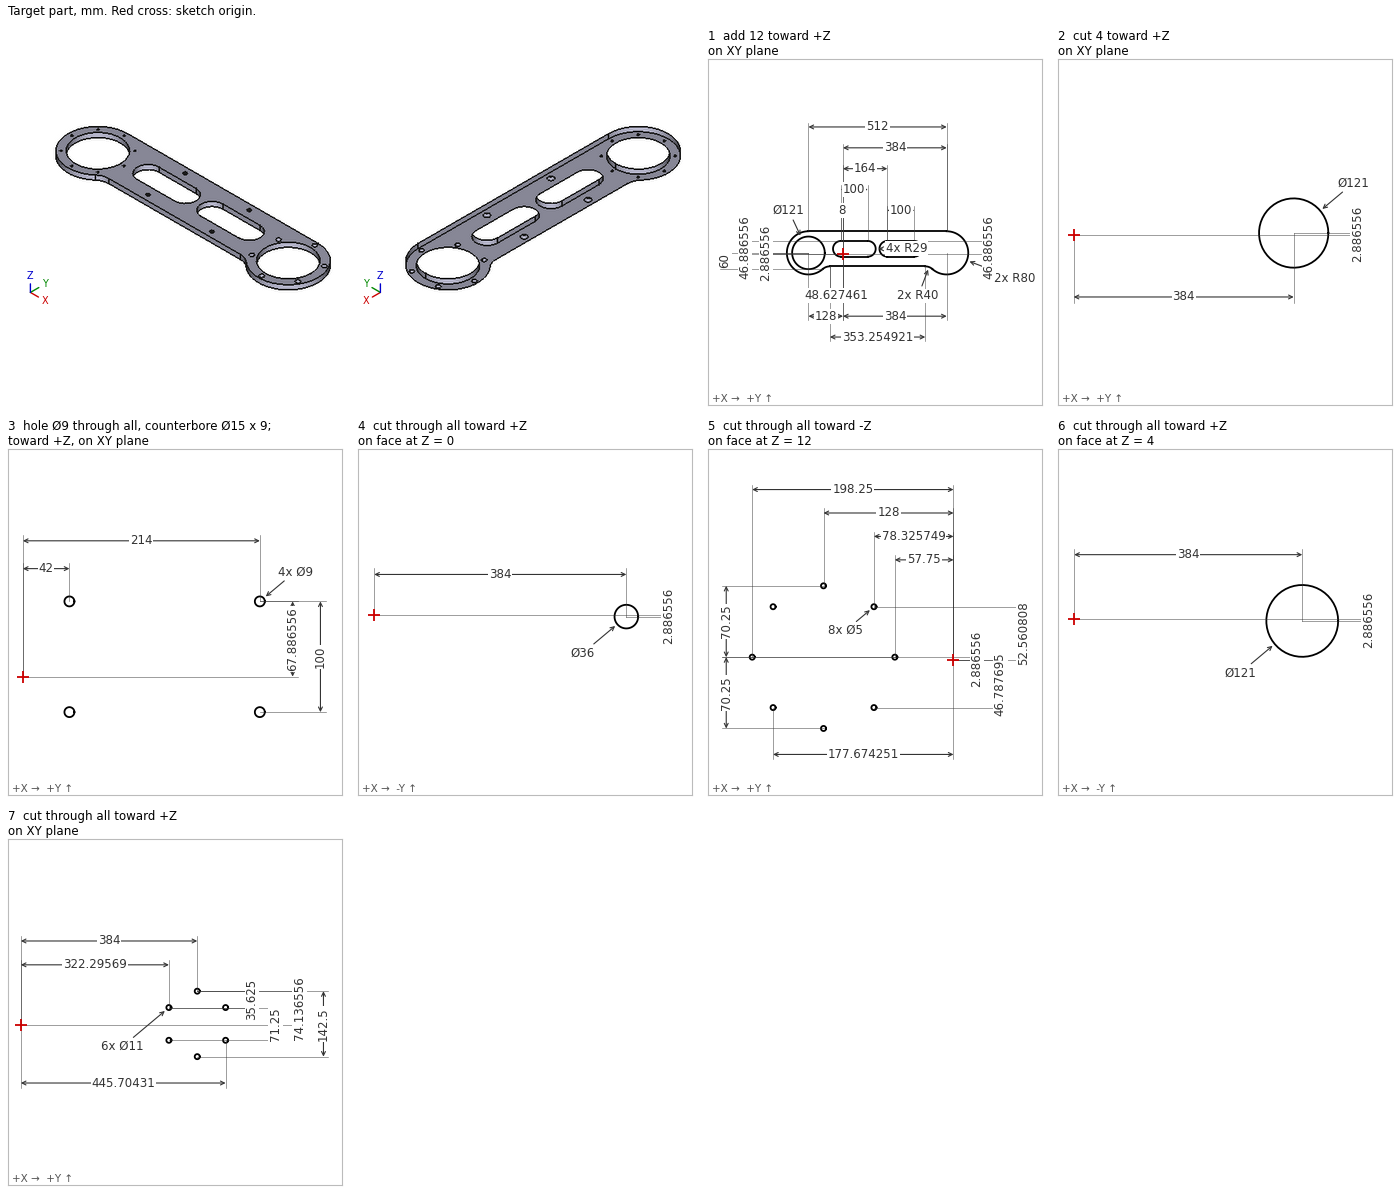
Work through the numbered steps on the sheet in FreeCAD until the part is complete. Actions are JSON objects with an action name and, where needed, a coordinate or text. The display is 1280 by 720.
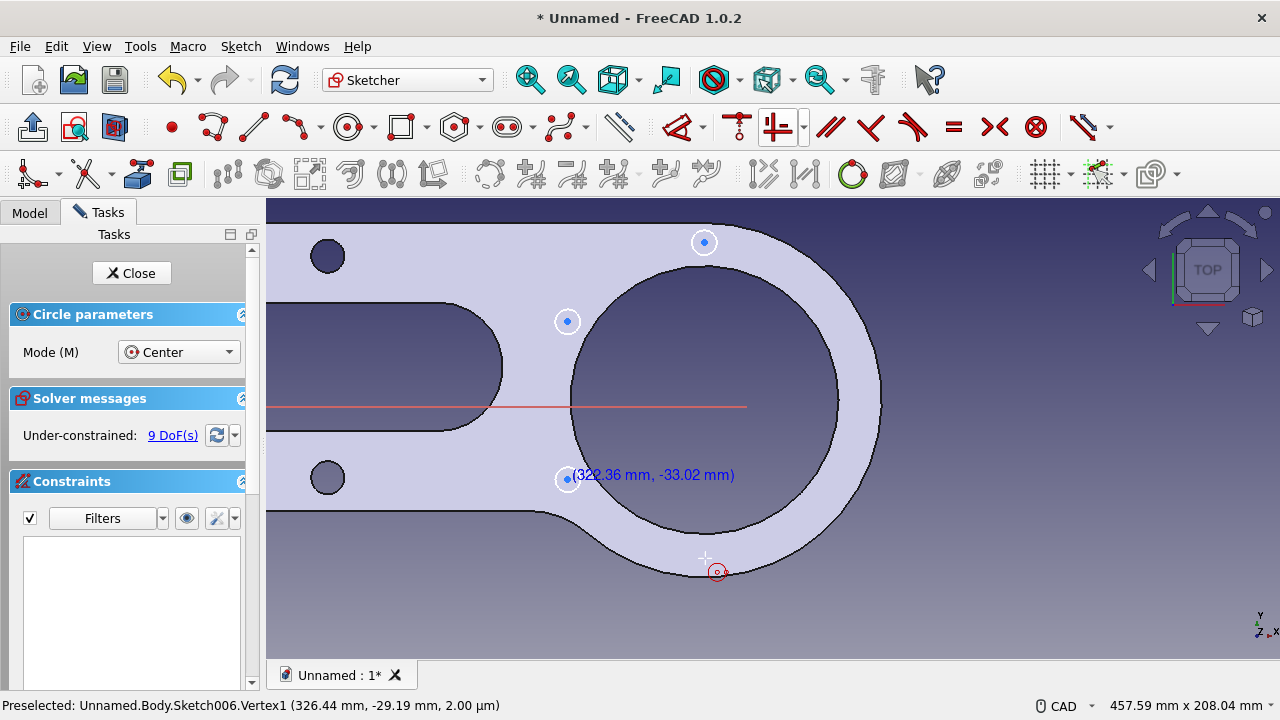
{"action": "left_click", "coordinate": [703, 557]}
{"action": "left_click", "coordinate": [723, 538]}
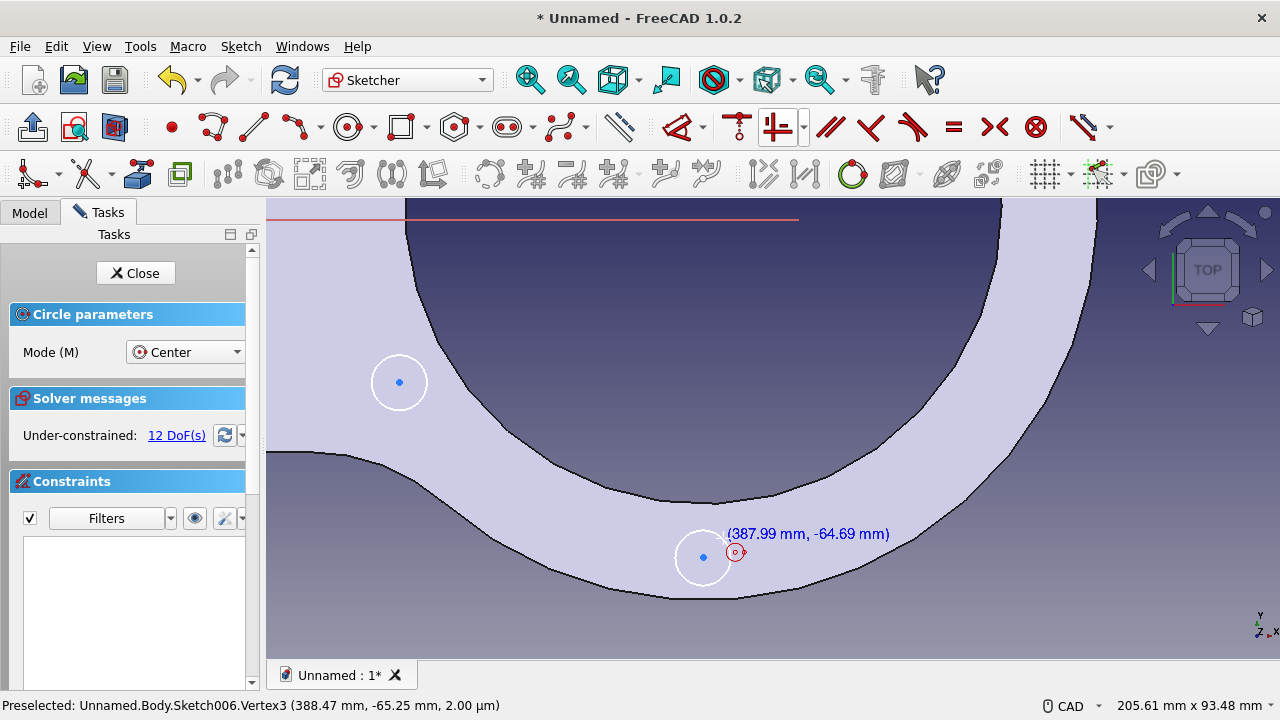
{"action": "left_click", "coordinate": [1008, 381]}
{"action": "left_click", "coordinate": [1027, 362]}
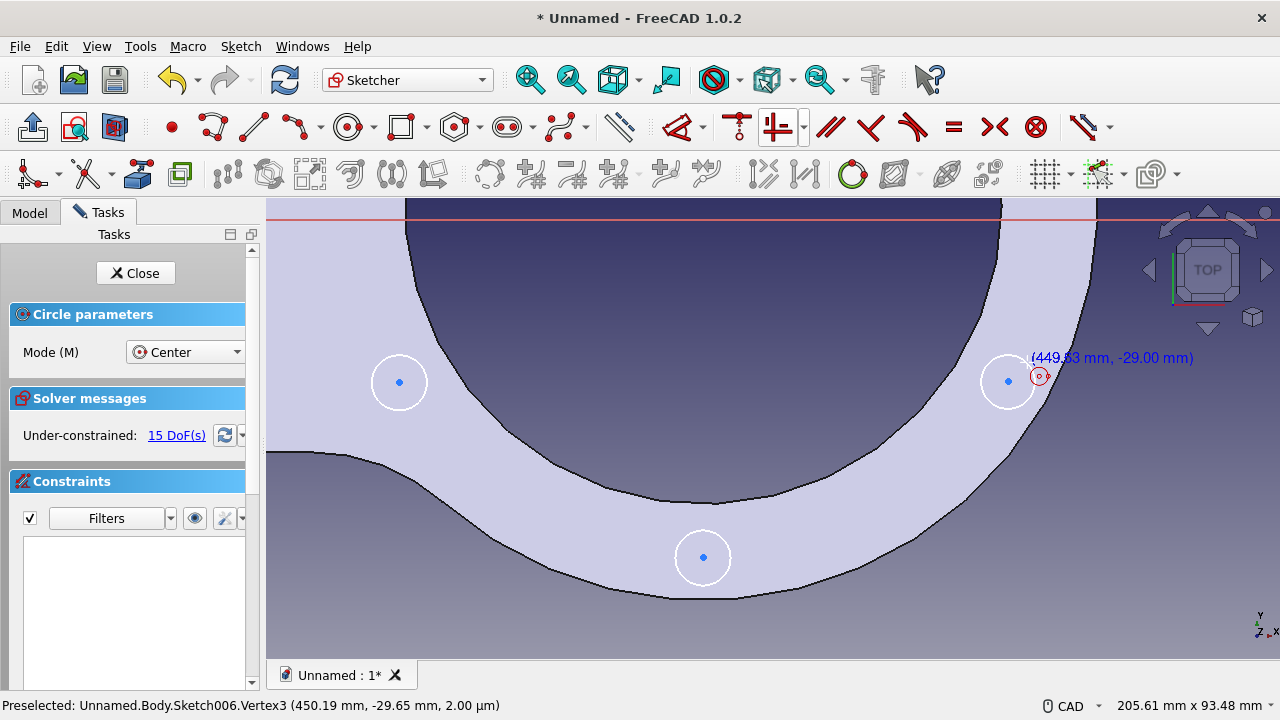
{"action": "scroll", "coordinate": [705, 558], "scroll_direction": "down", "scroll_amount": 5}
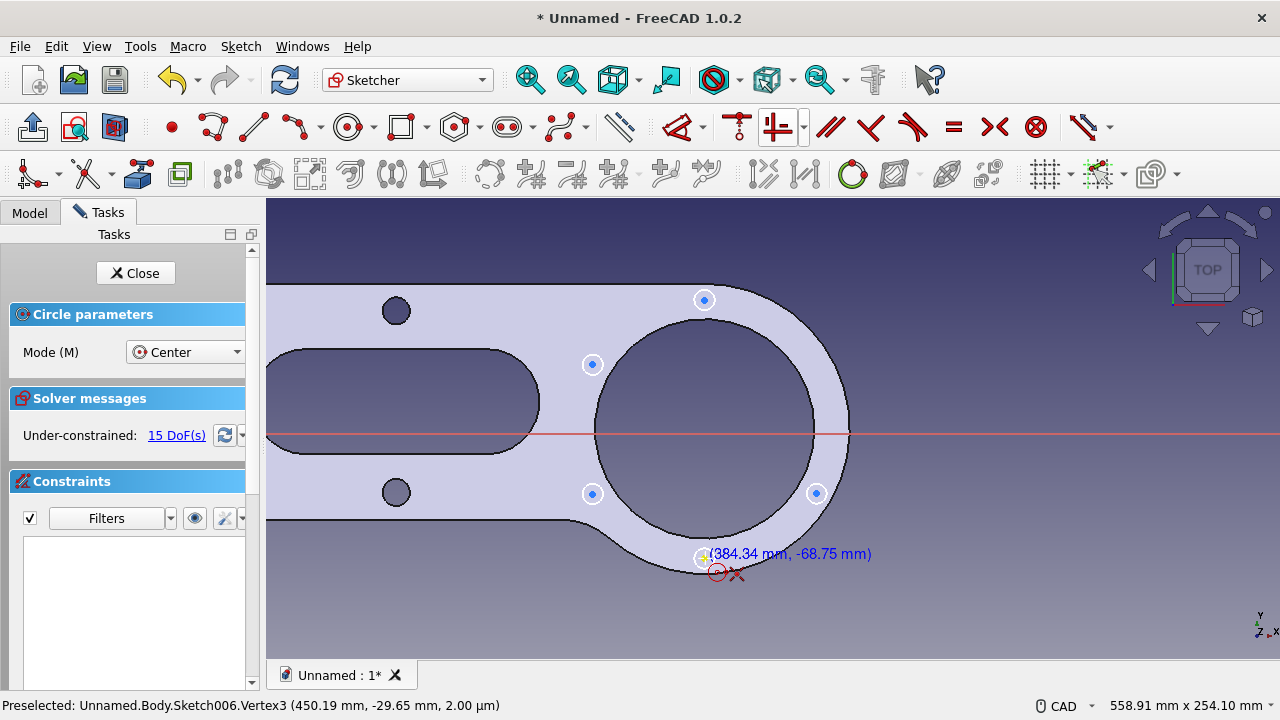
{"action": "scroll", "coordinate": [817, 364], "scroll_direction": "up", "scroll_amount": 5}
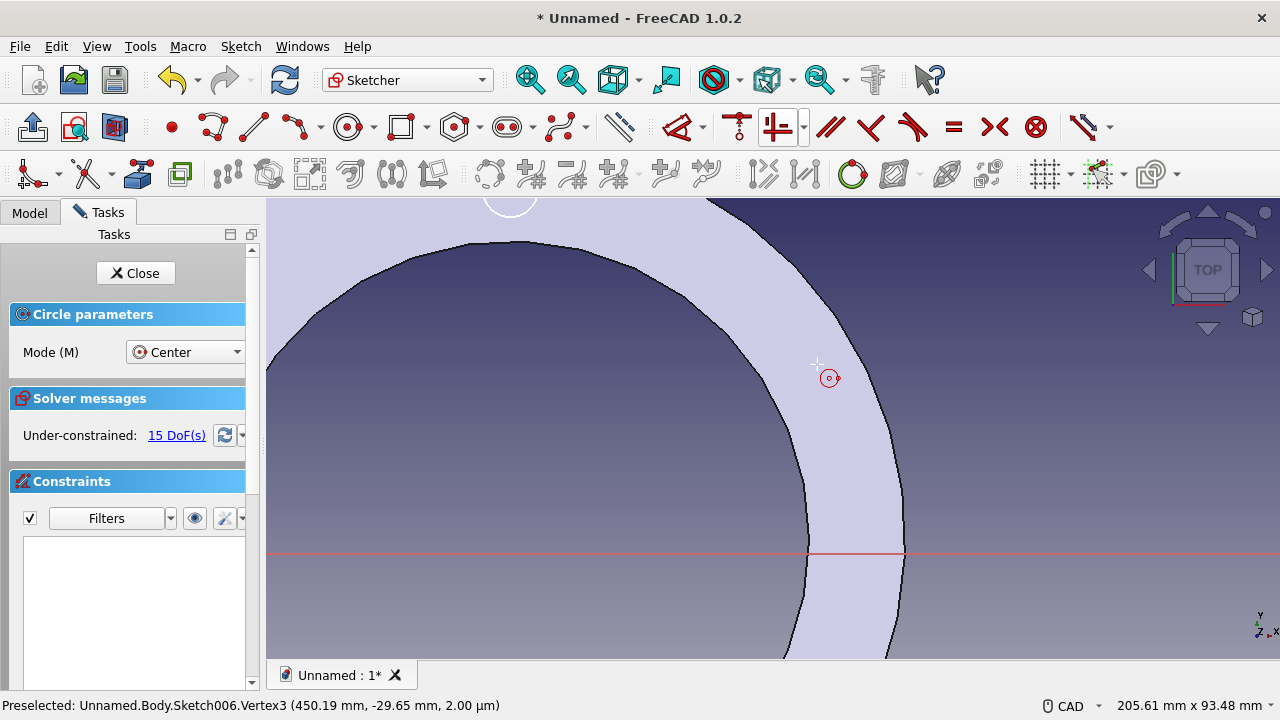
{"action": "left_click", "coordinate": [815, 364]}
{"action": "left_click", "coordinate": [834, 345]}
{"action": "key", "text": "Escape"}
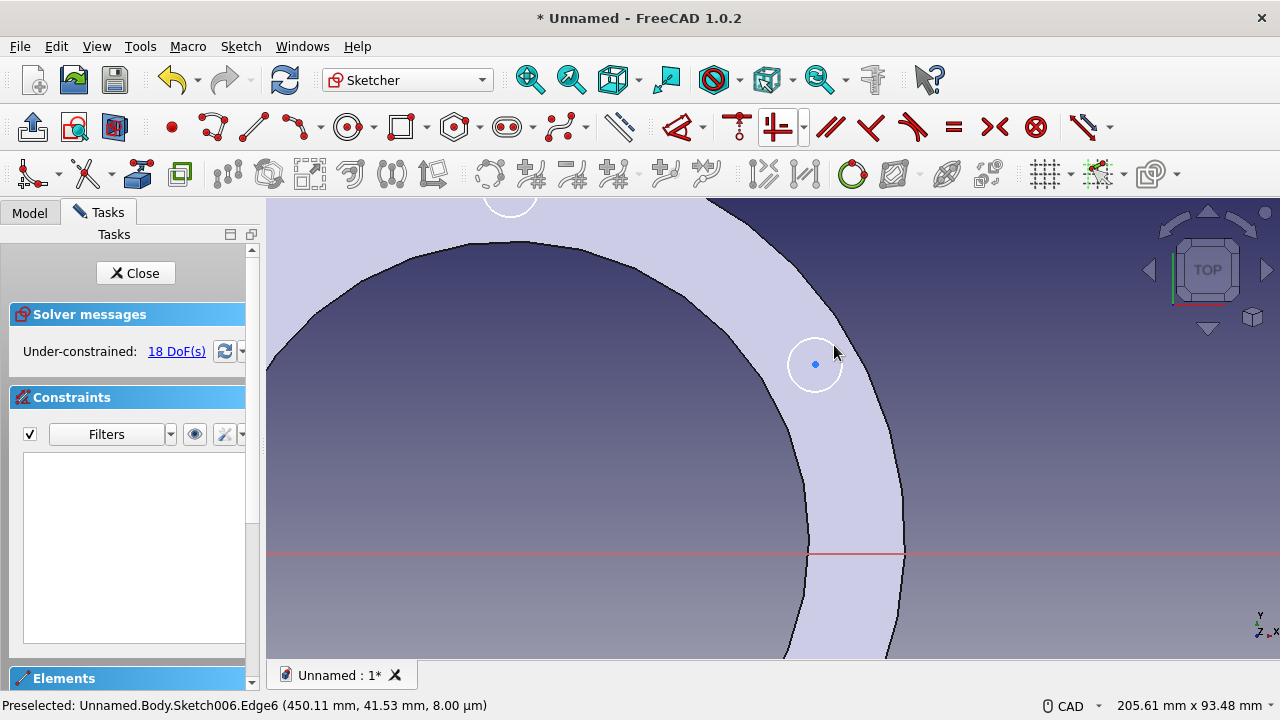
{"action": "scroll", "coordinate": [817, 364], "scroll_direction": "down", "scroll_amount": 5}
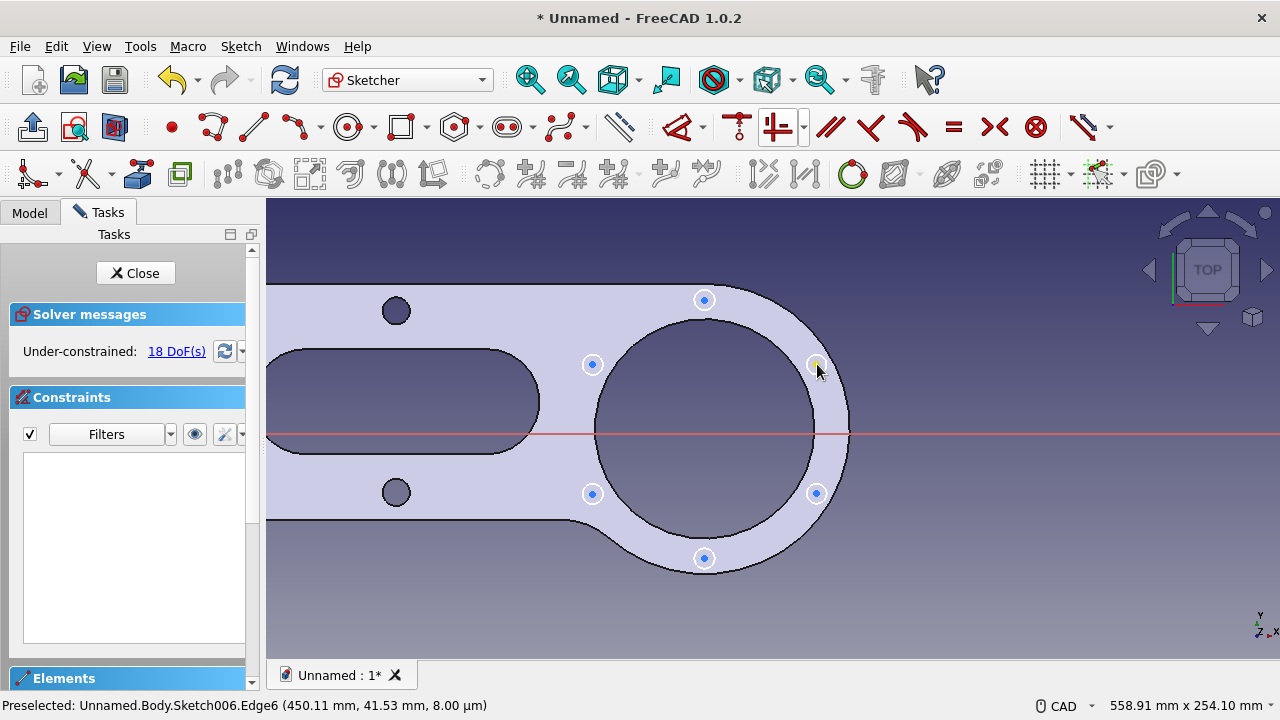
{"action": "scroll", "coordinate": [712, 293], "scroll_direction": "up", "scroll_amount": 2}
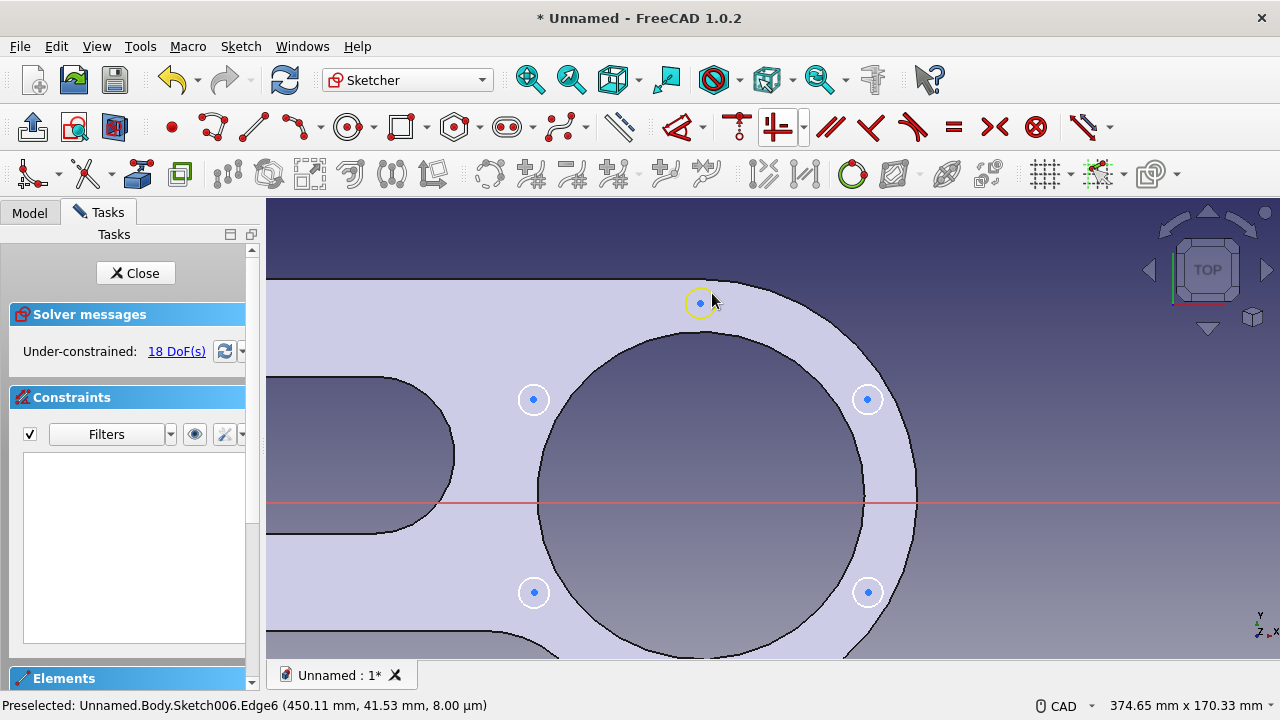
{"action": "left_click", "coordinate": [711, 293]}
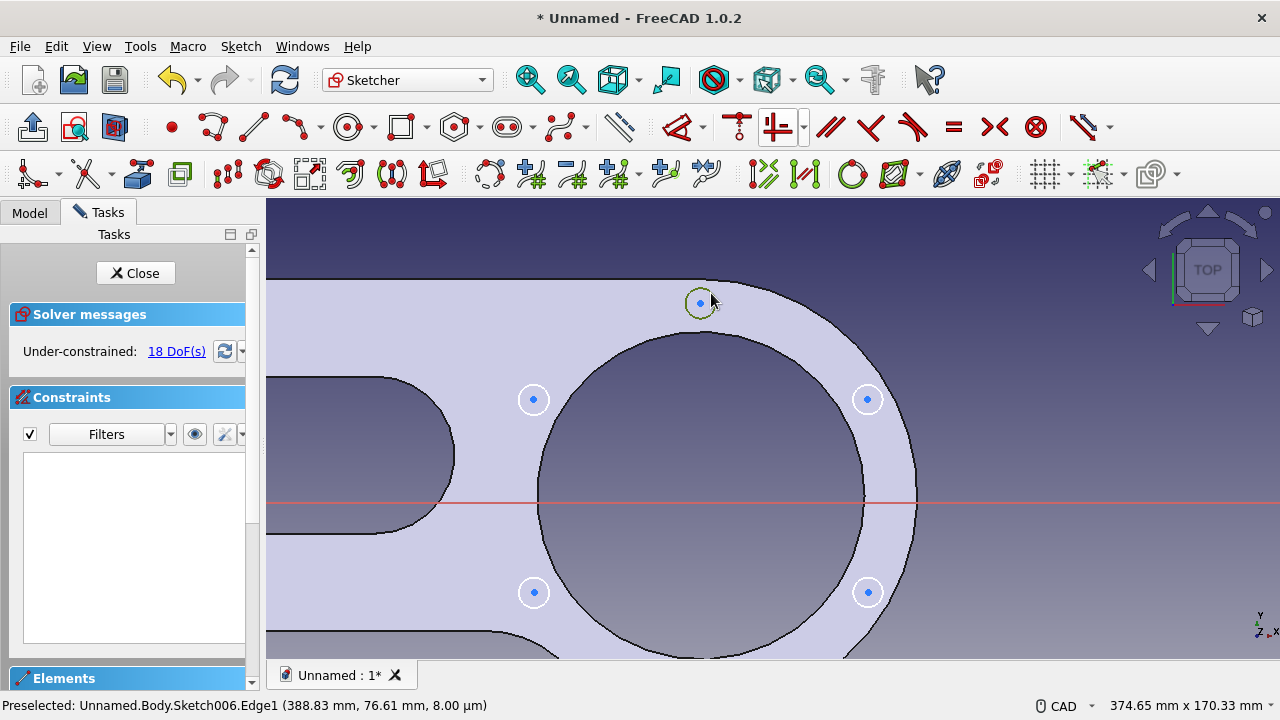
{"action": "left_click", "coordinate": [544, 389]}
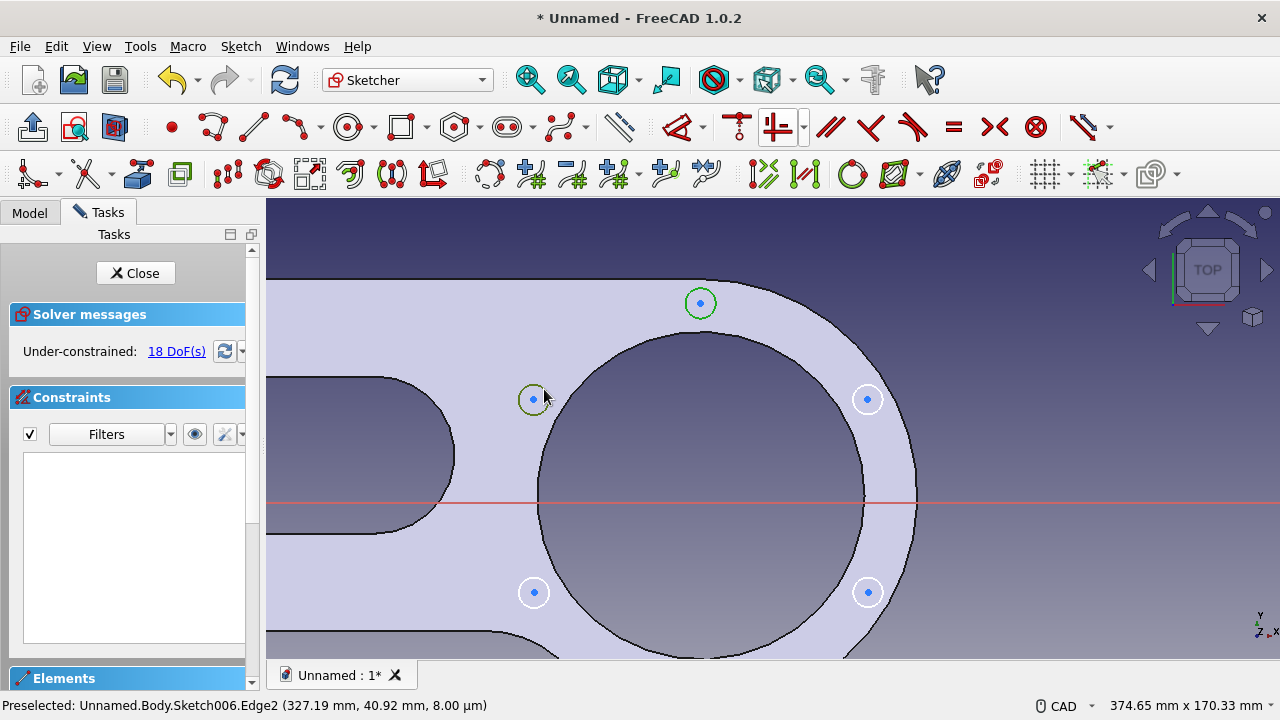
{"action": "left_click", "coordinate": [545, 582]}